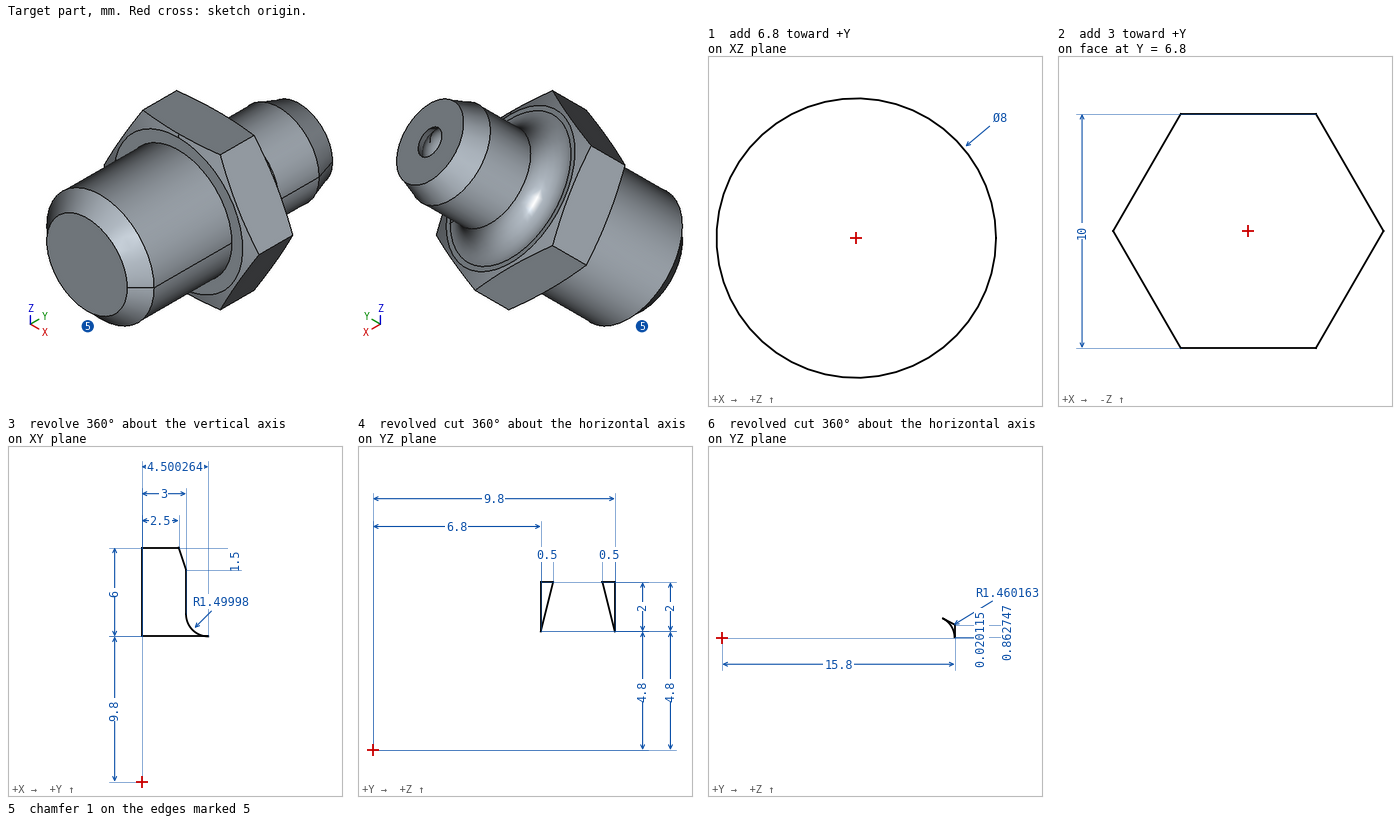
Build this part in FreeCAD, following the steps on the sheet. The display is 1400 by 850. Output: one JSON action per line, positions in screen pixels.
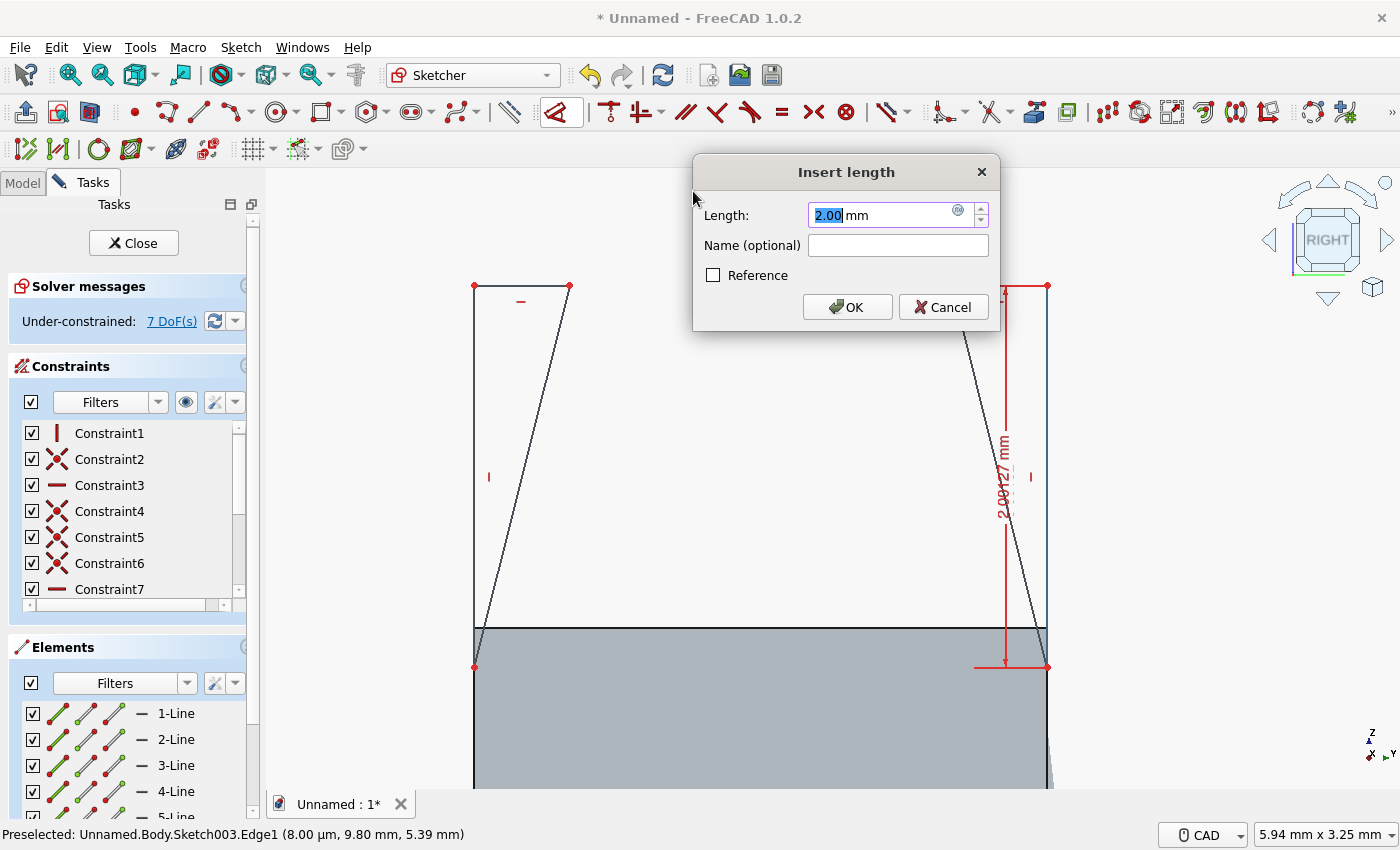
{"action": "type", "text": "2"}
{"action": "key", "text": "Return"}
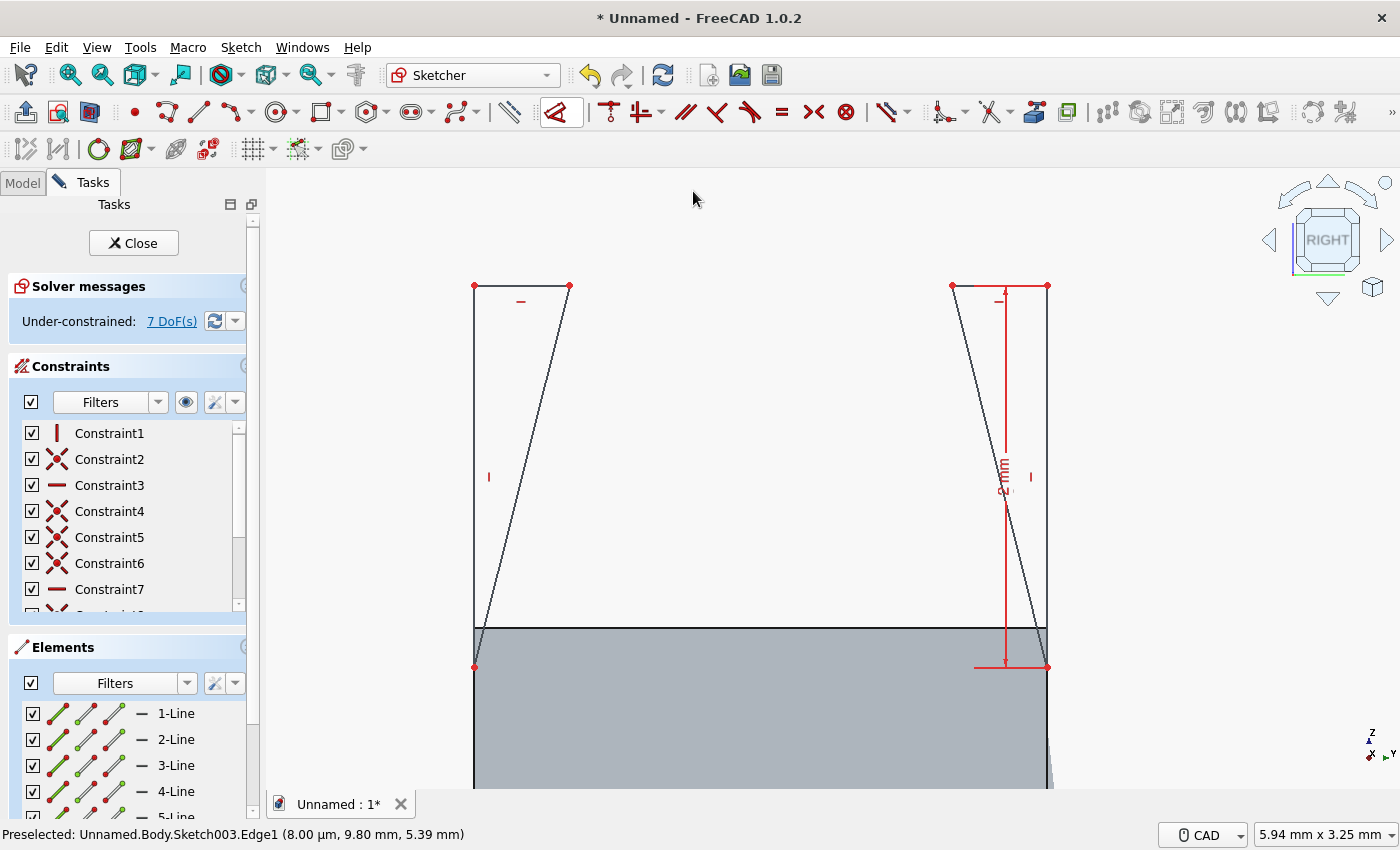
{"action": "left_click", "coordinate": [474, 401]}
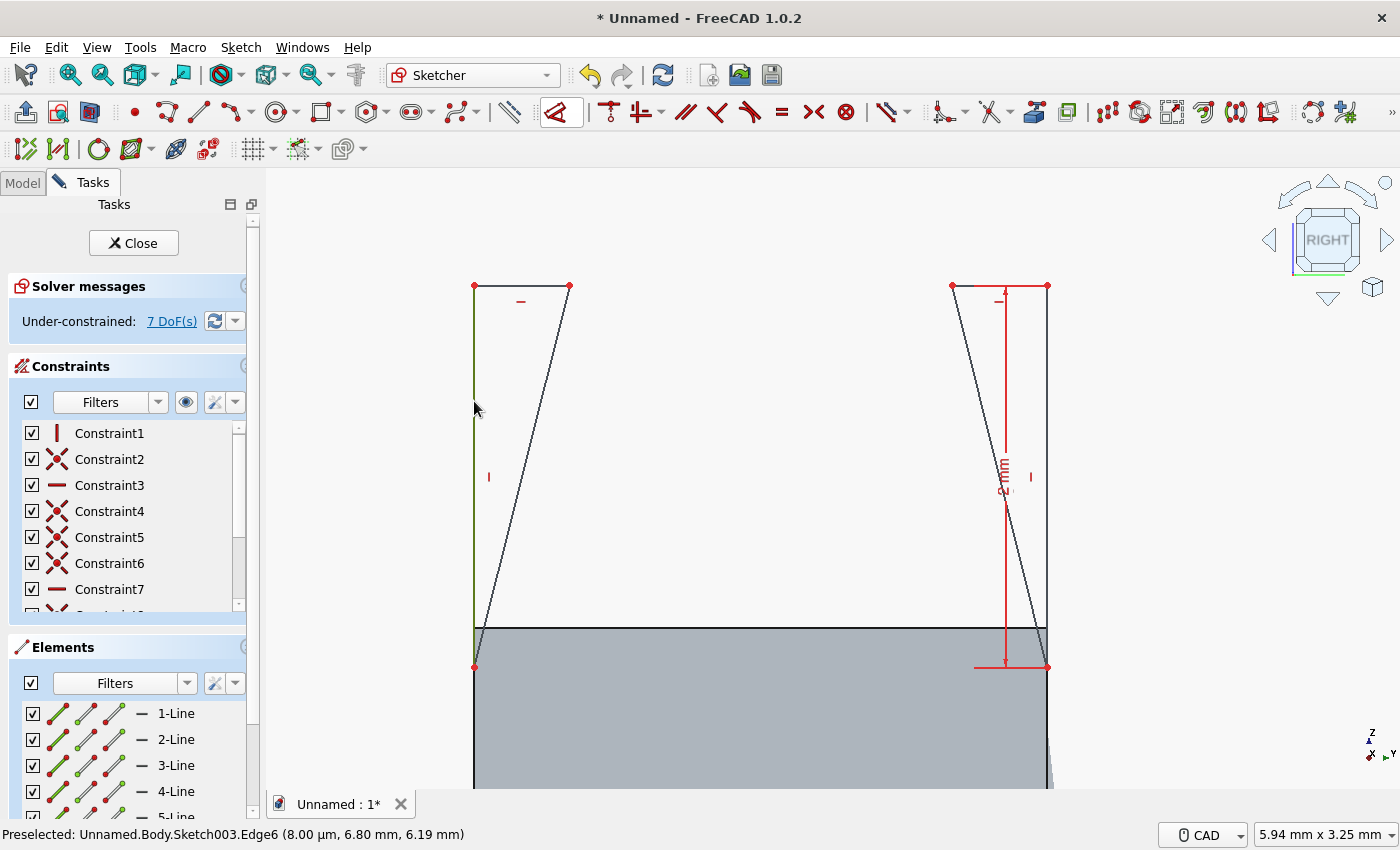
{"action": "key", "text": "i"}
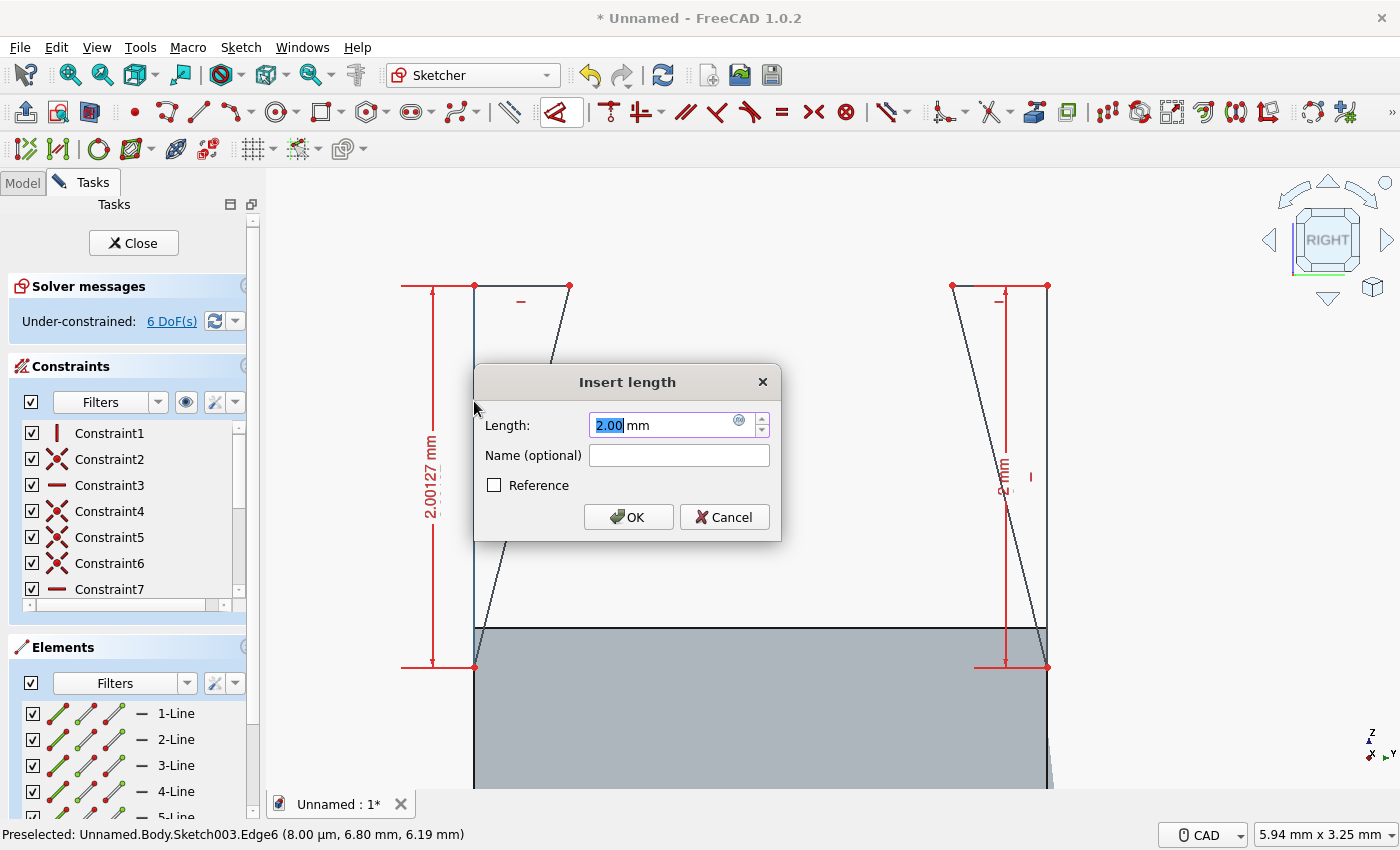
{"action": "type", "text": "2"}
{"action": "key", "text": "Return"}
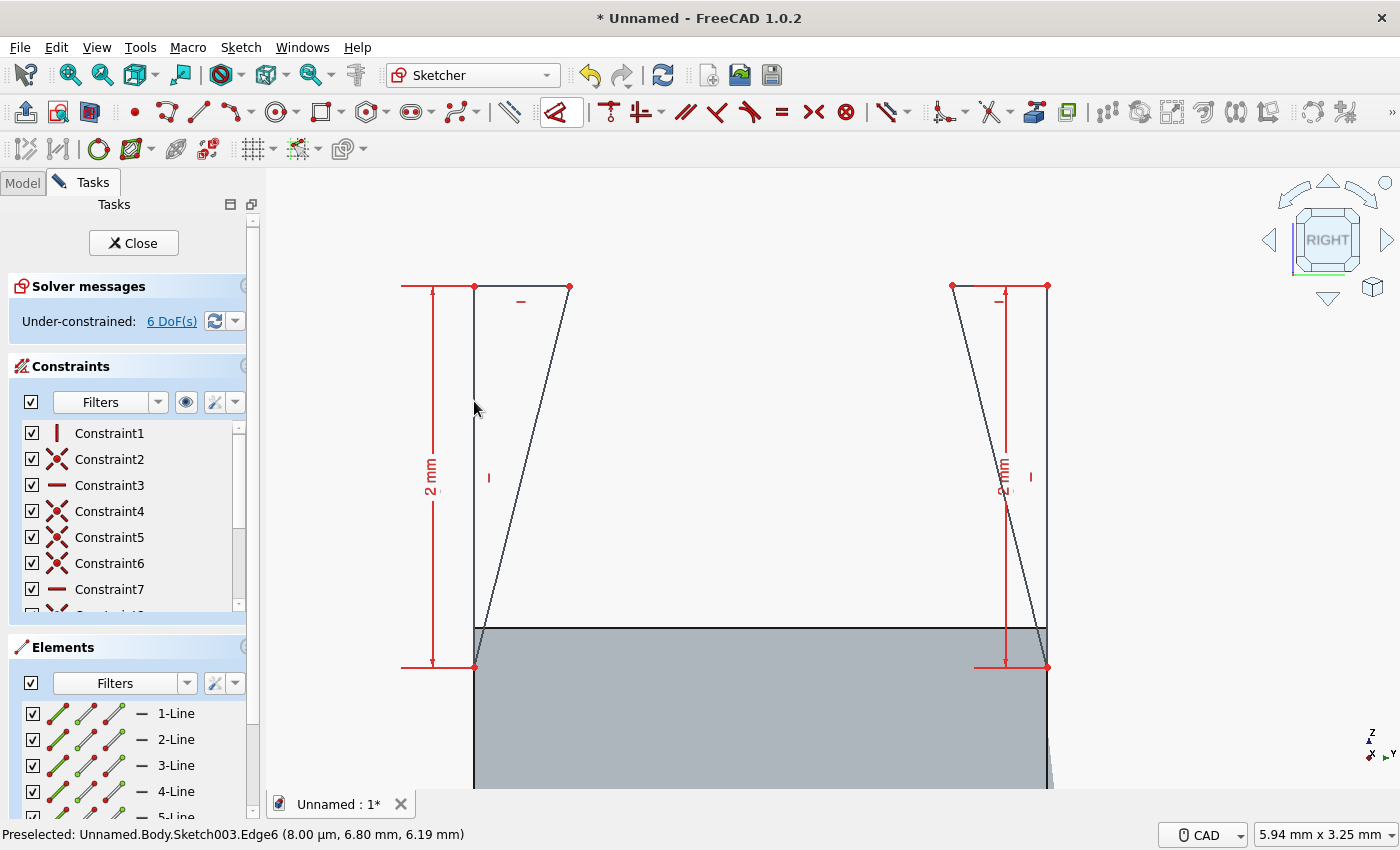
{"action": "left_click", "coordinate": [1019, 286]}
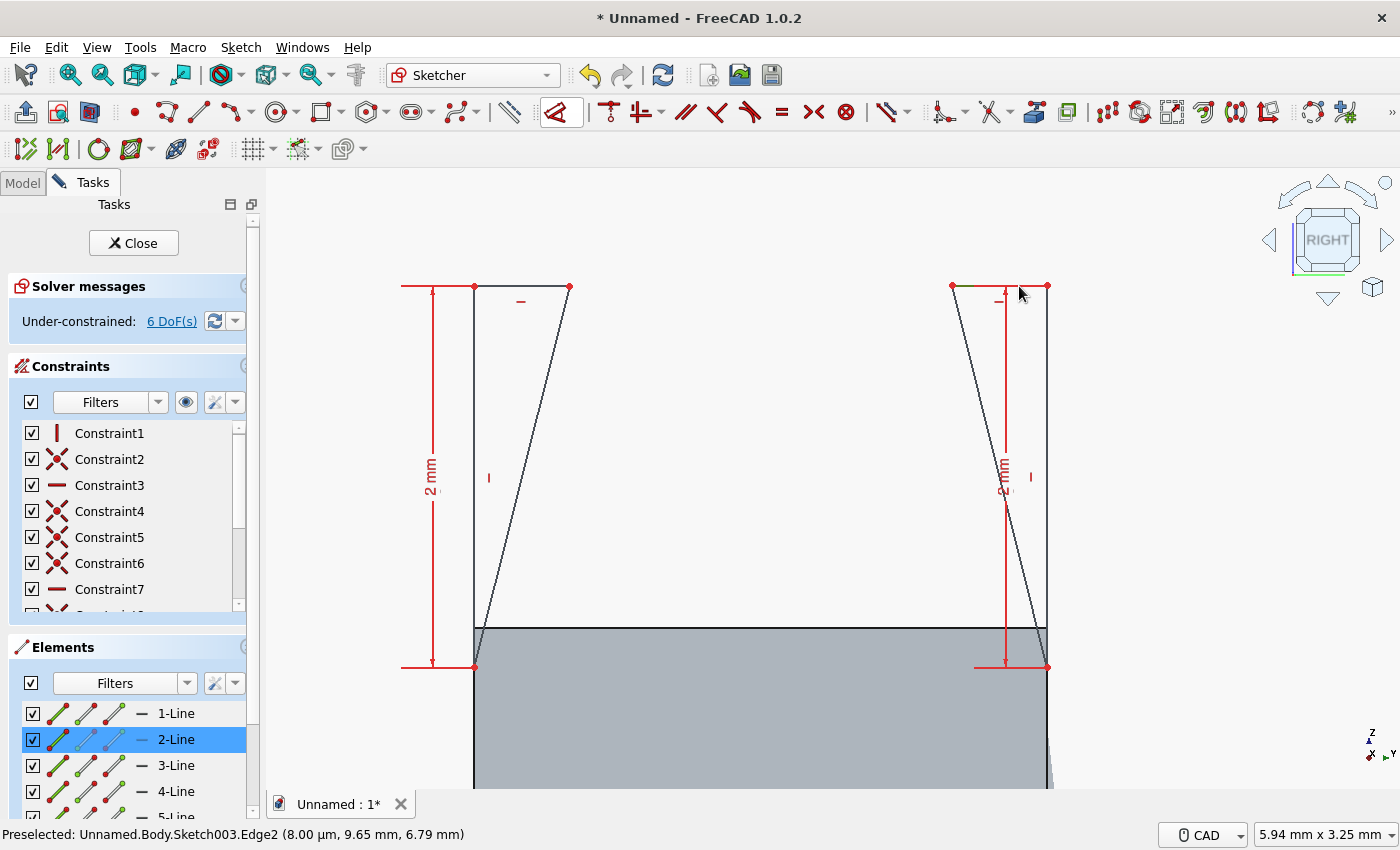
{"action": "key", "text": "l"}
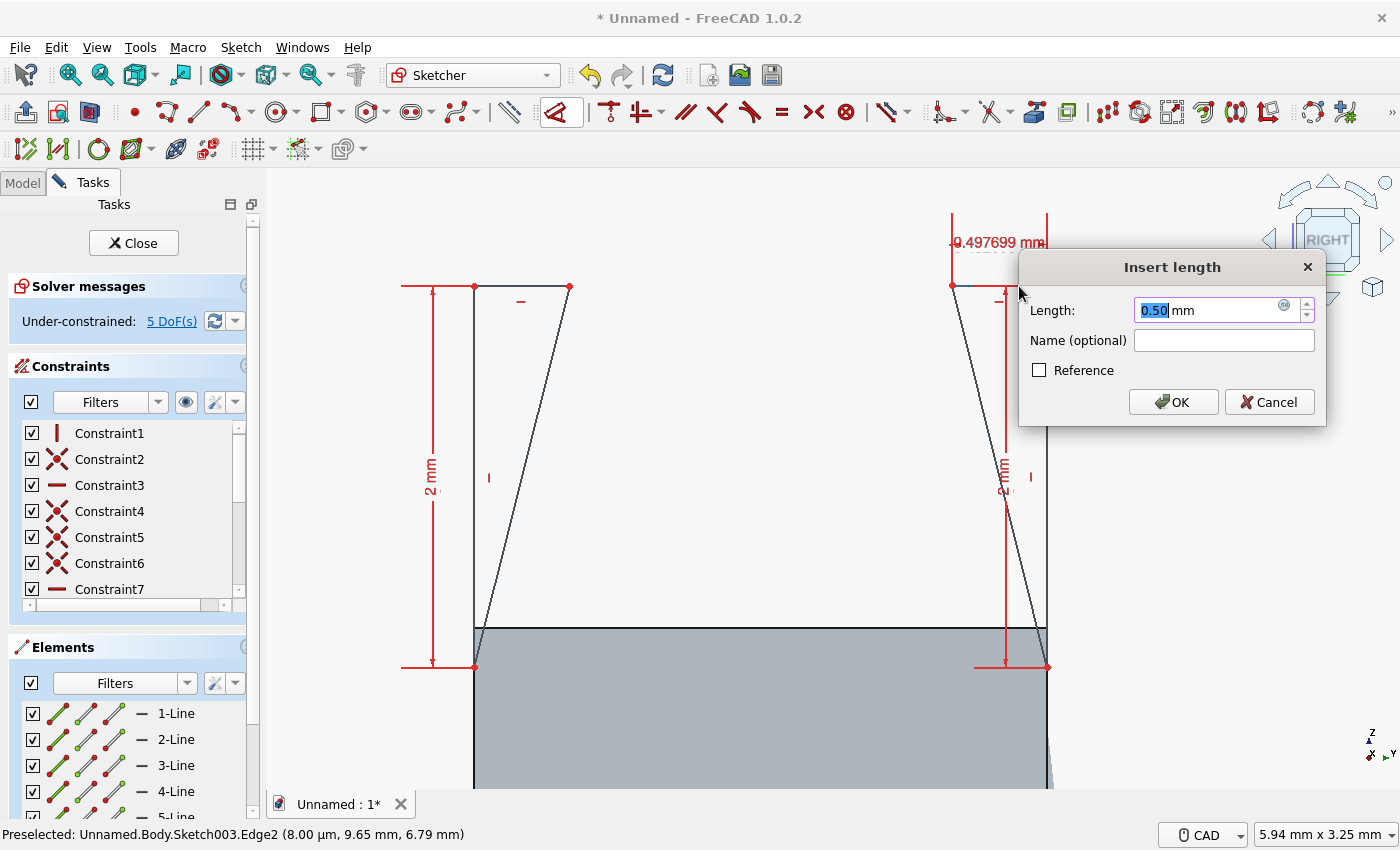
{"action": "type", "text": "0.5"}
{"action": "key", "text": "Return"}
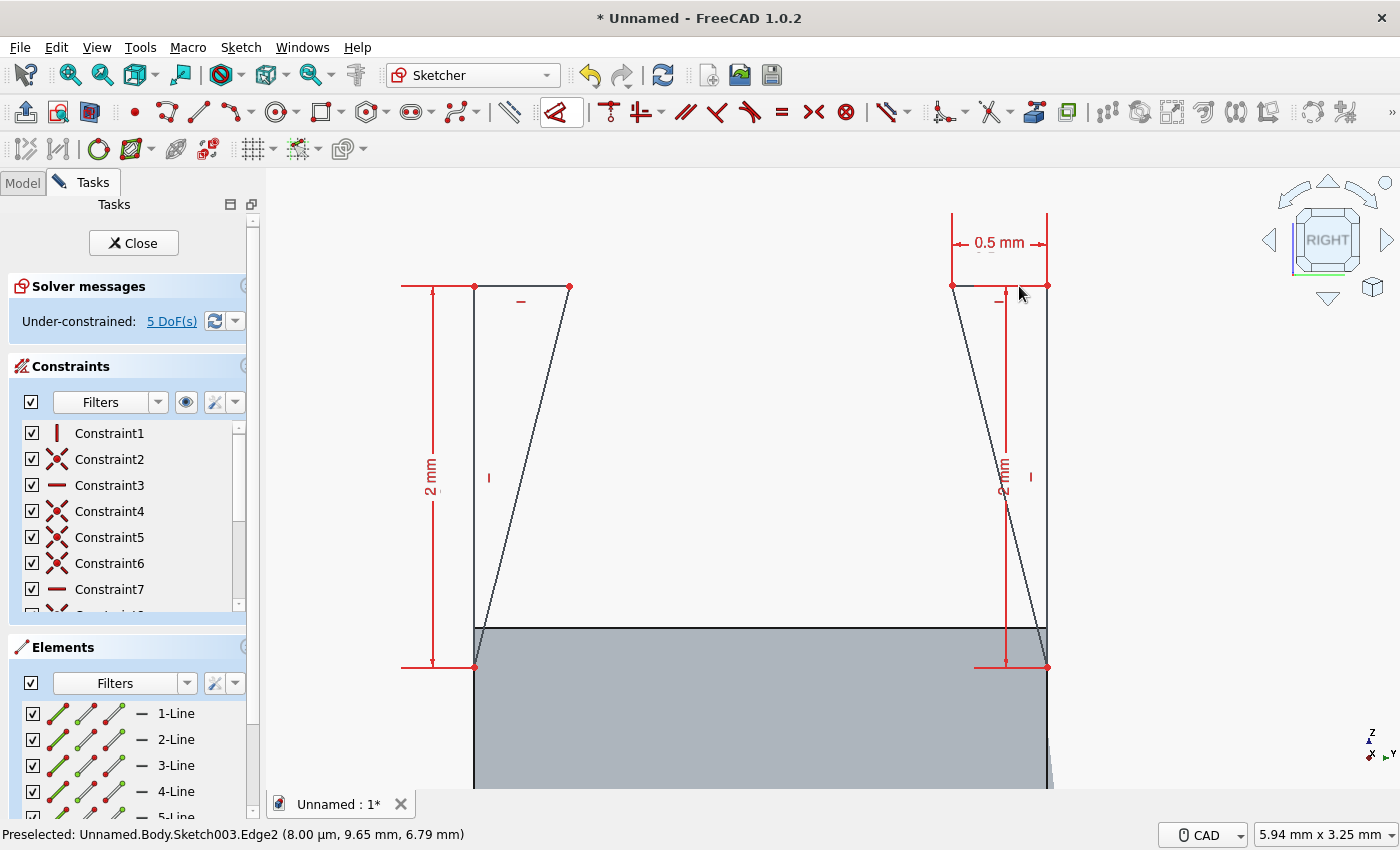
{"action": "left_click", "coordinate": [541, 286]}